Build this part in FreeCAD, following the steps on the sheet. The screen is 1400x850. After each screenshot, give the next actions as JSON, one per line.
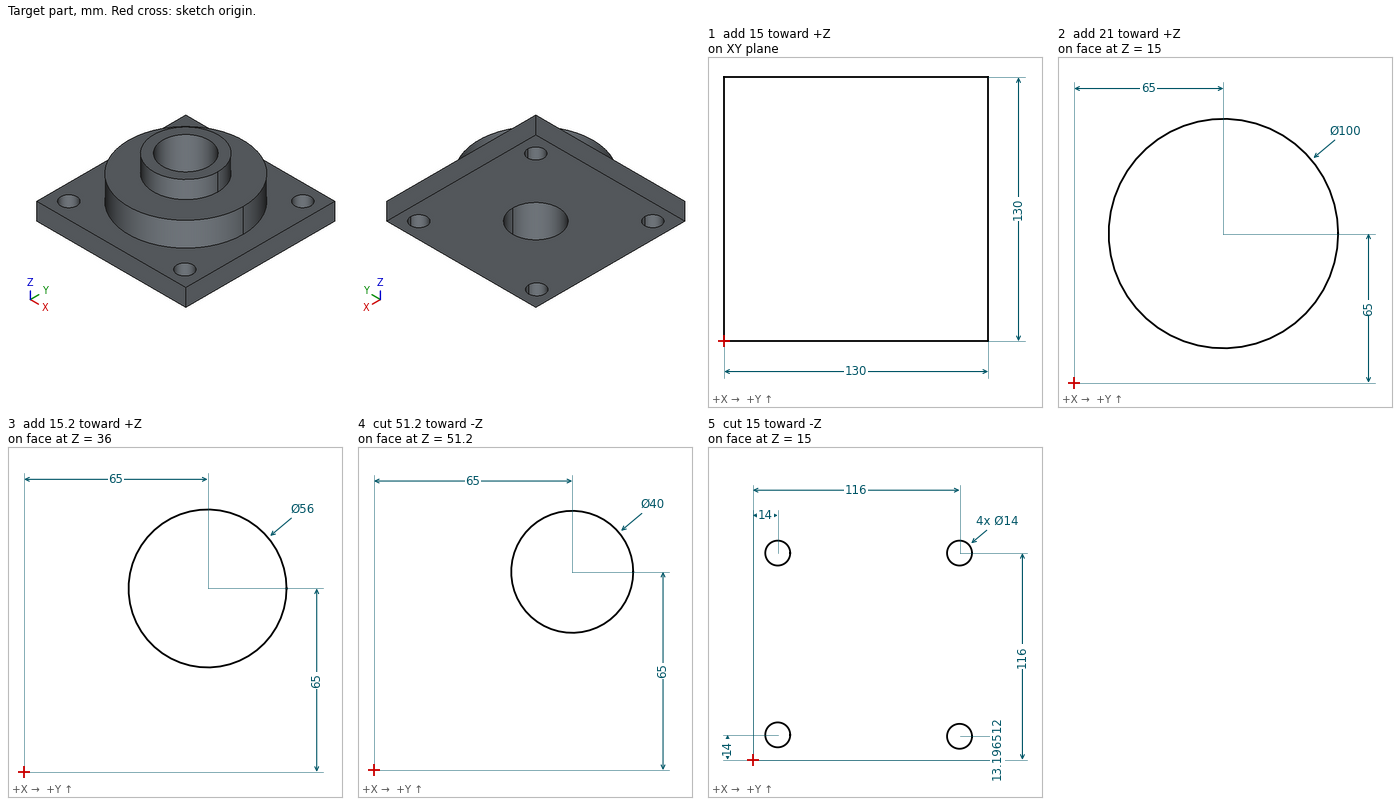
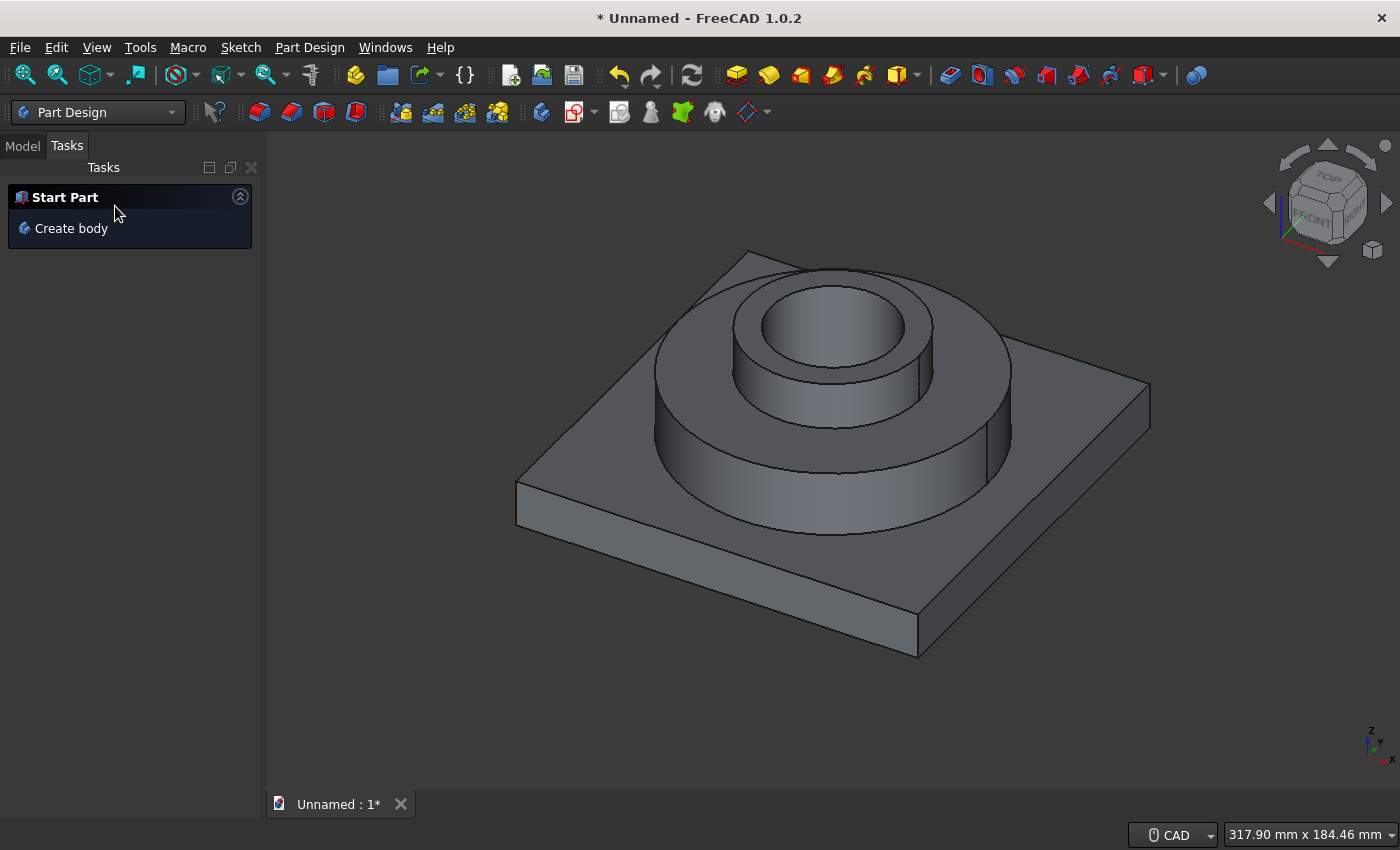
{"action": "left_click", "coordinate": [1104, 390]}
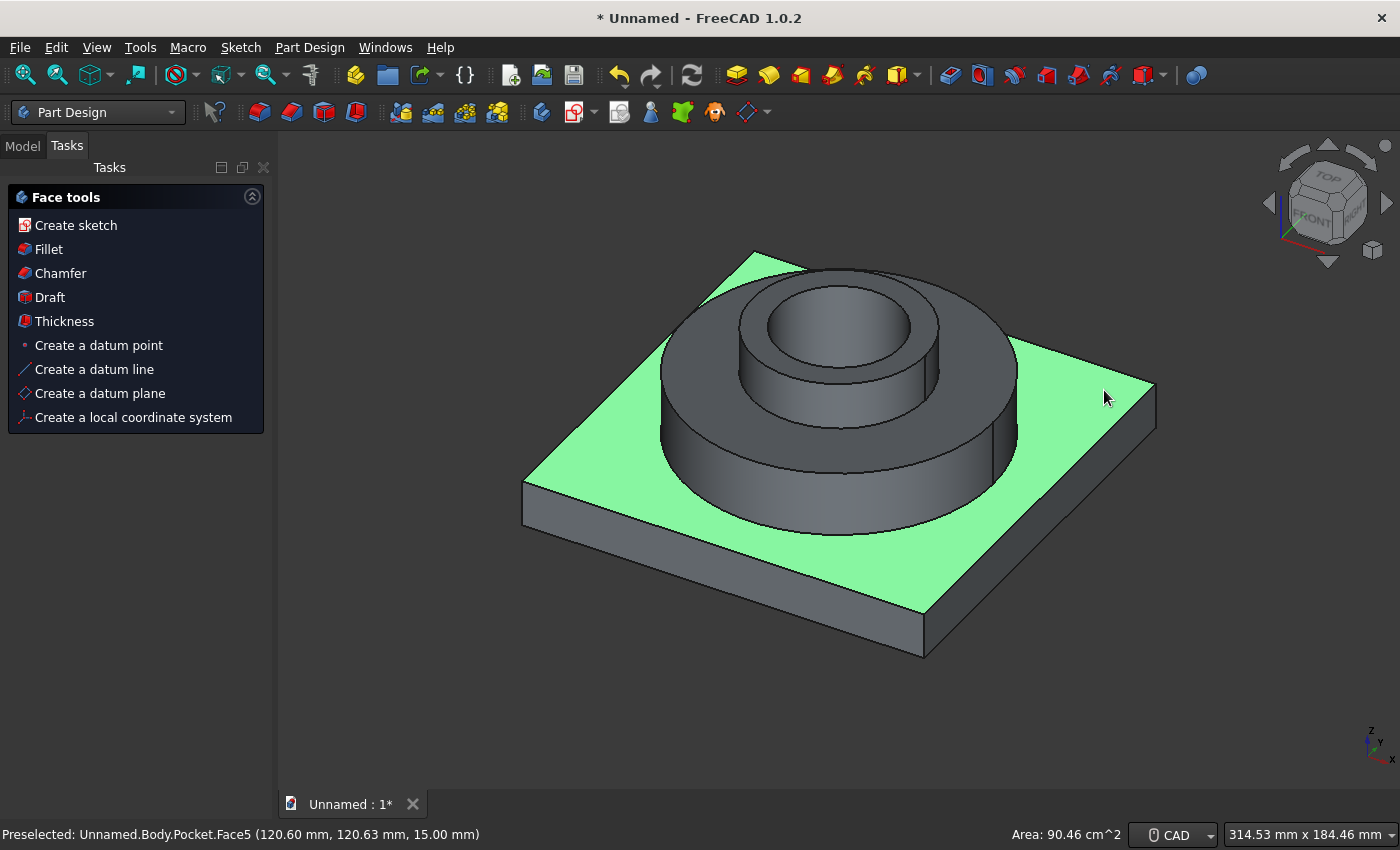
{"action": "left_click", "coordinate": [574, 112]}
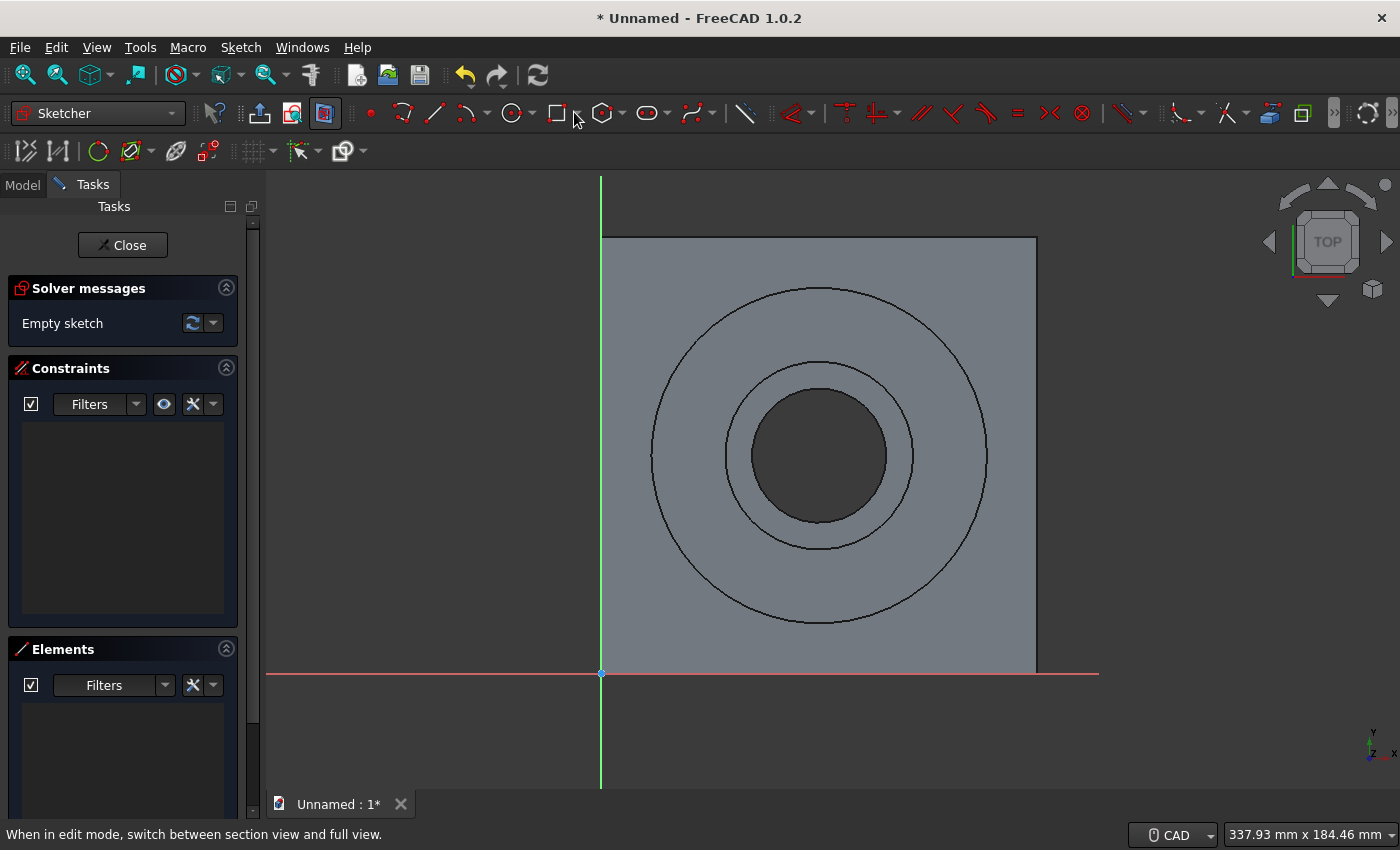
{"action": "left_click", "coordinate": [326, 114]}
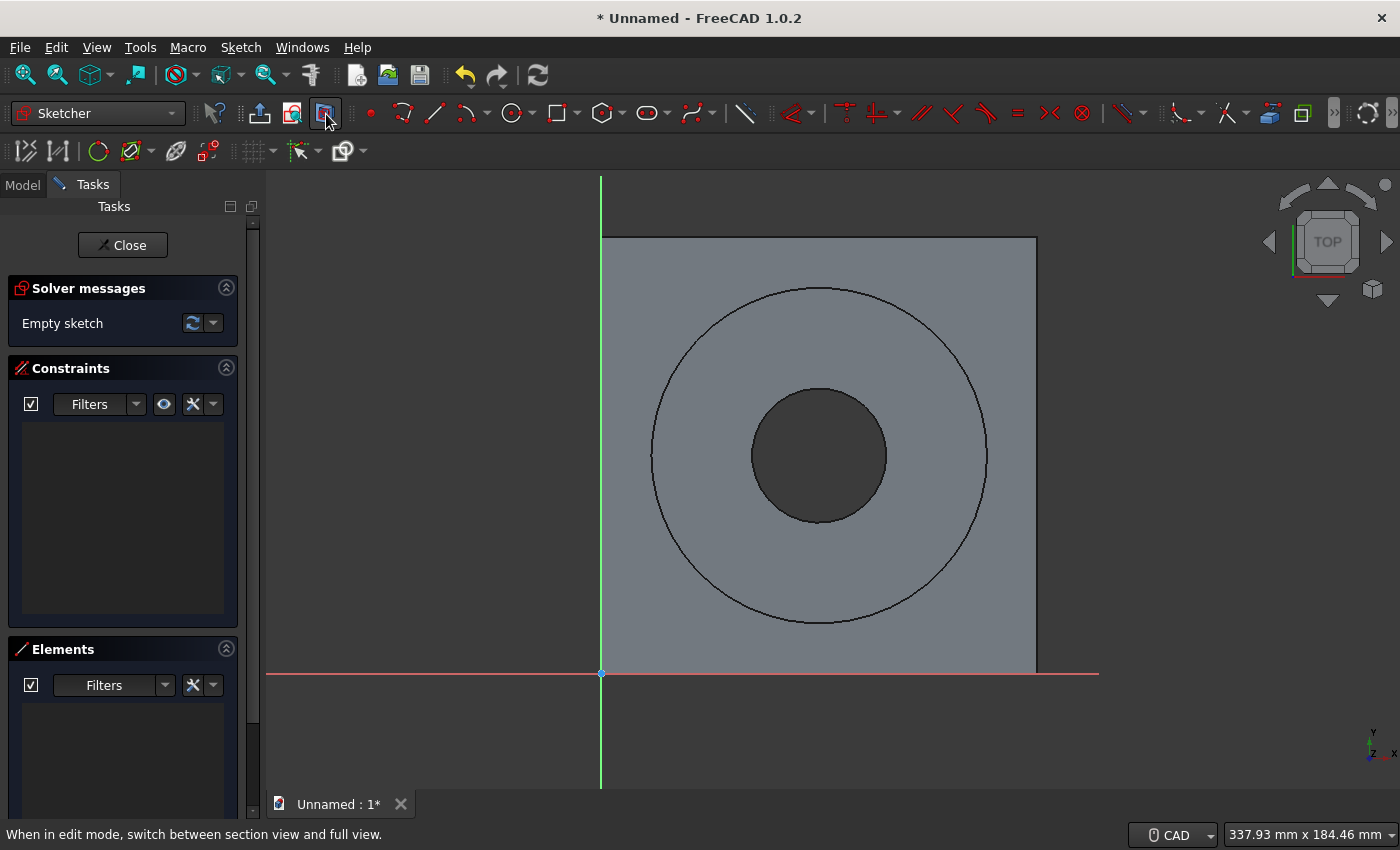
{"action": "key", "text": "g c"}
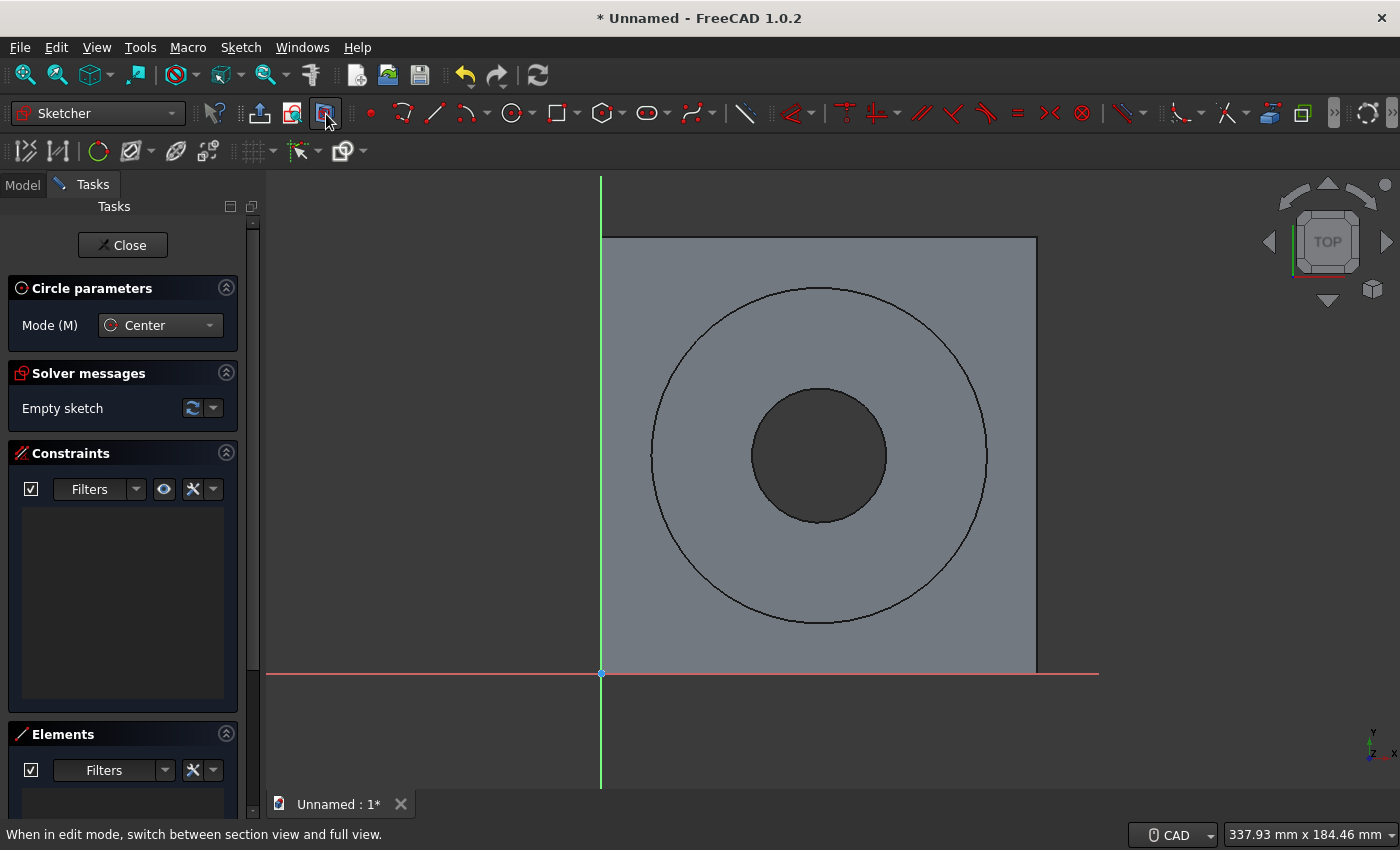
{"action": "left_click", "coordinate": [990, 284]}
{"action": "mouse_move", "coordinate": [1007, 268]}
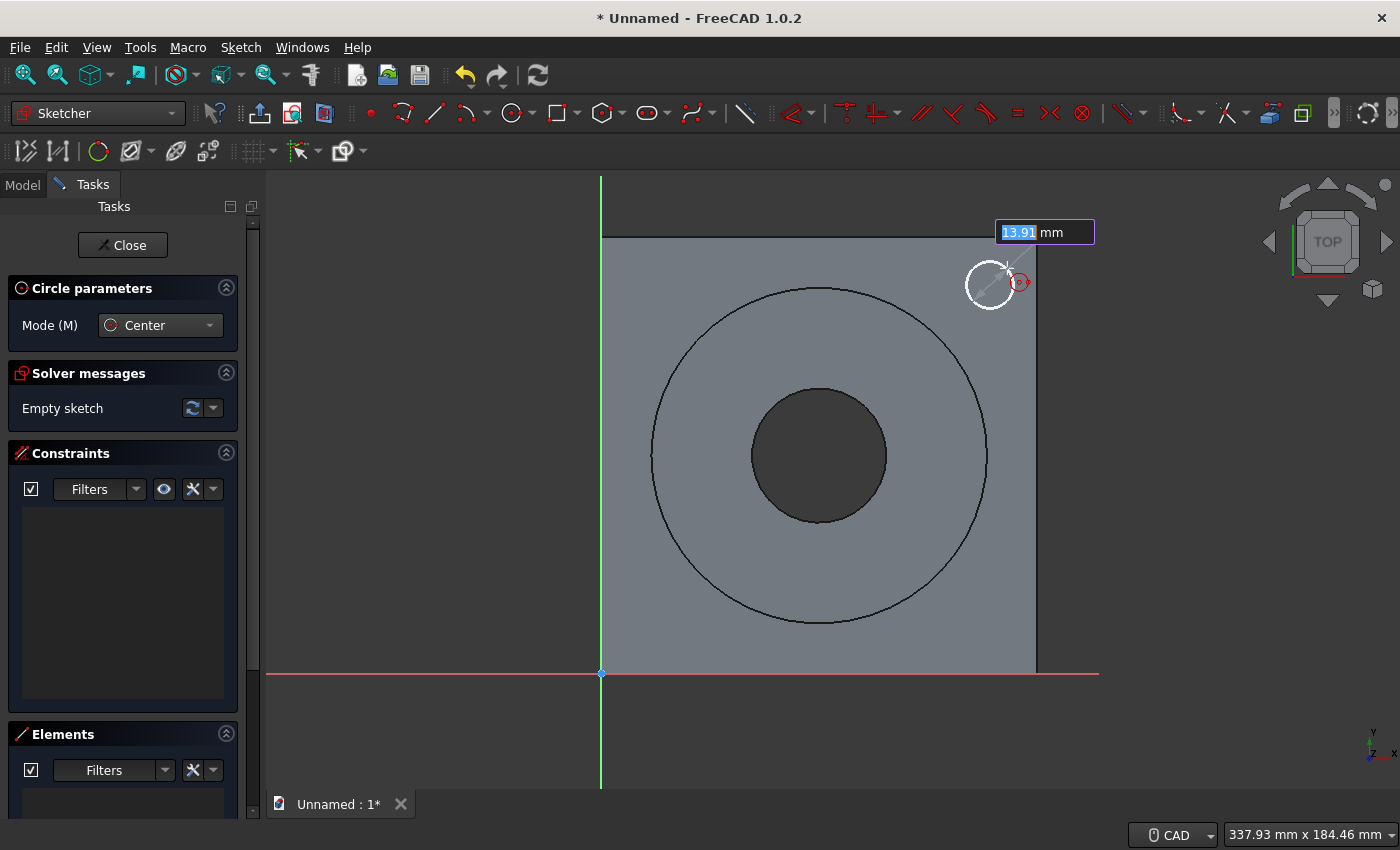
{"action": "type", "text": "14"}
{"action": "key", "text": "Return"}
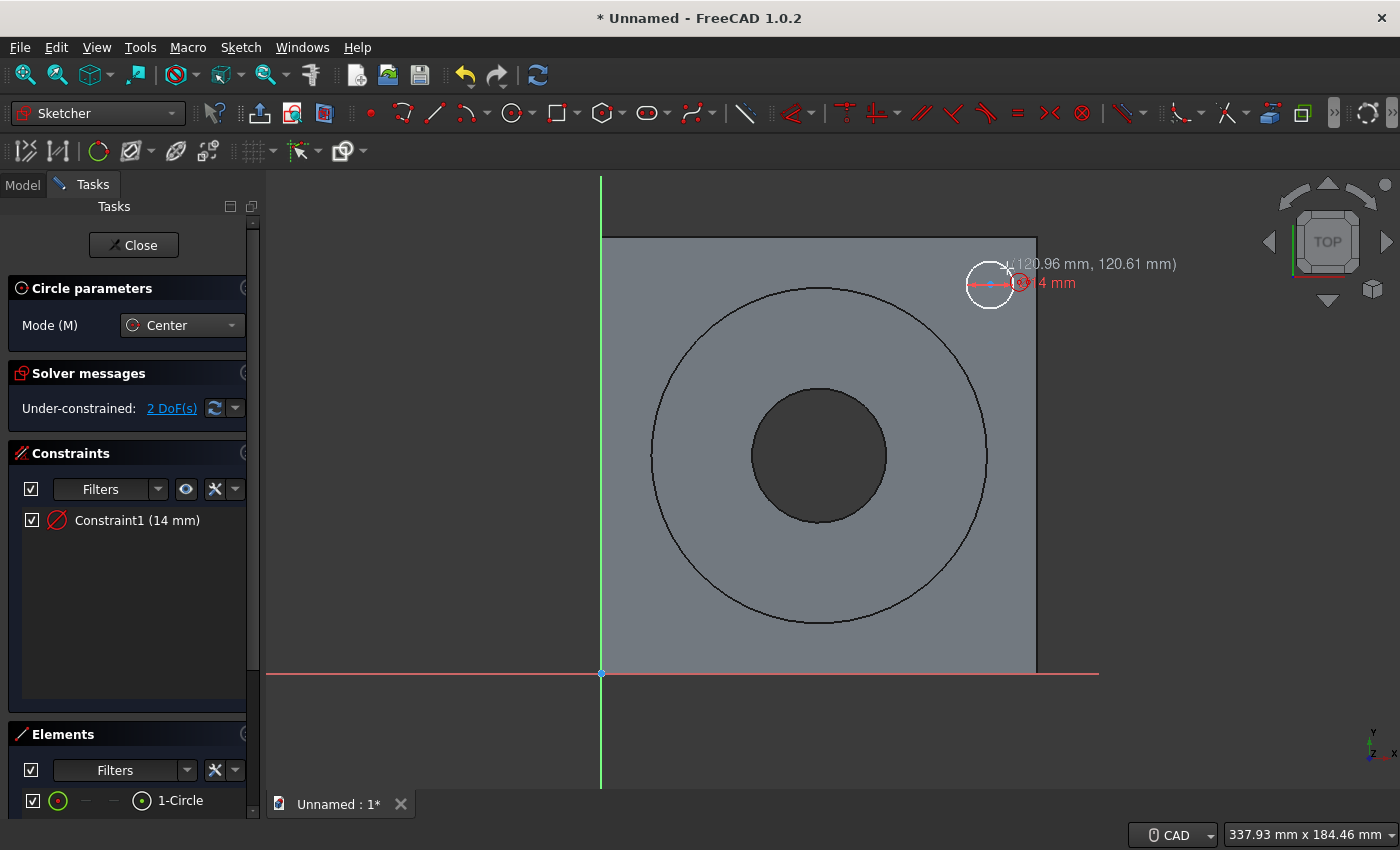
{"action": "left_click", "coordinate": [648, 284]}
{"action": "mouse_move", "coordinate": [665, 268]}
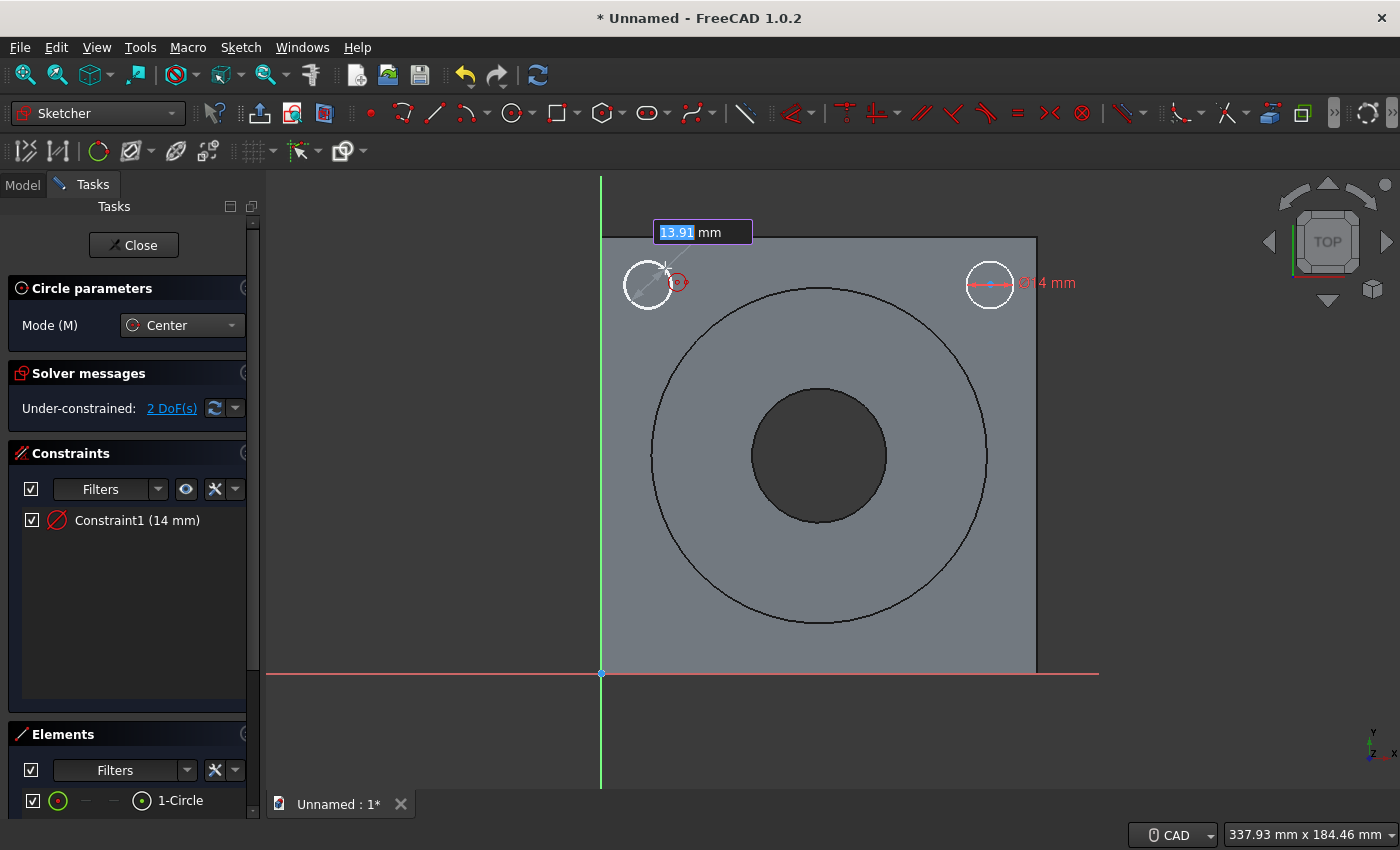
{"action": "type", "text": "14"}
{"action": "key", "text": "Return"}